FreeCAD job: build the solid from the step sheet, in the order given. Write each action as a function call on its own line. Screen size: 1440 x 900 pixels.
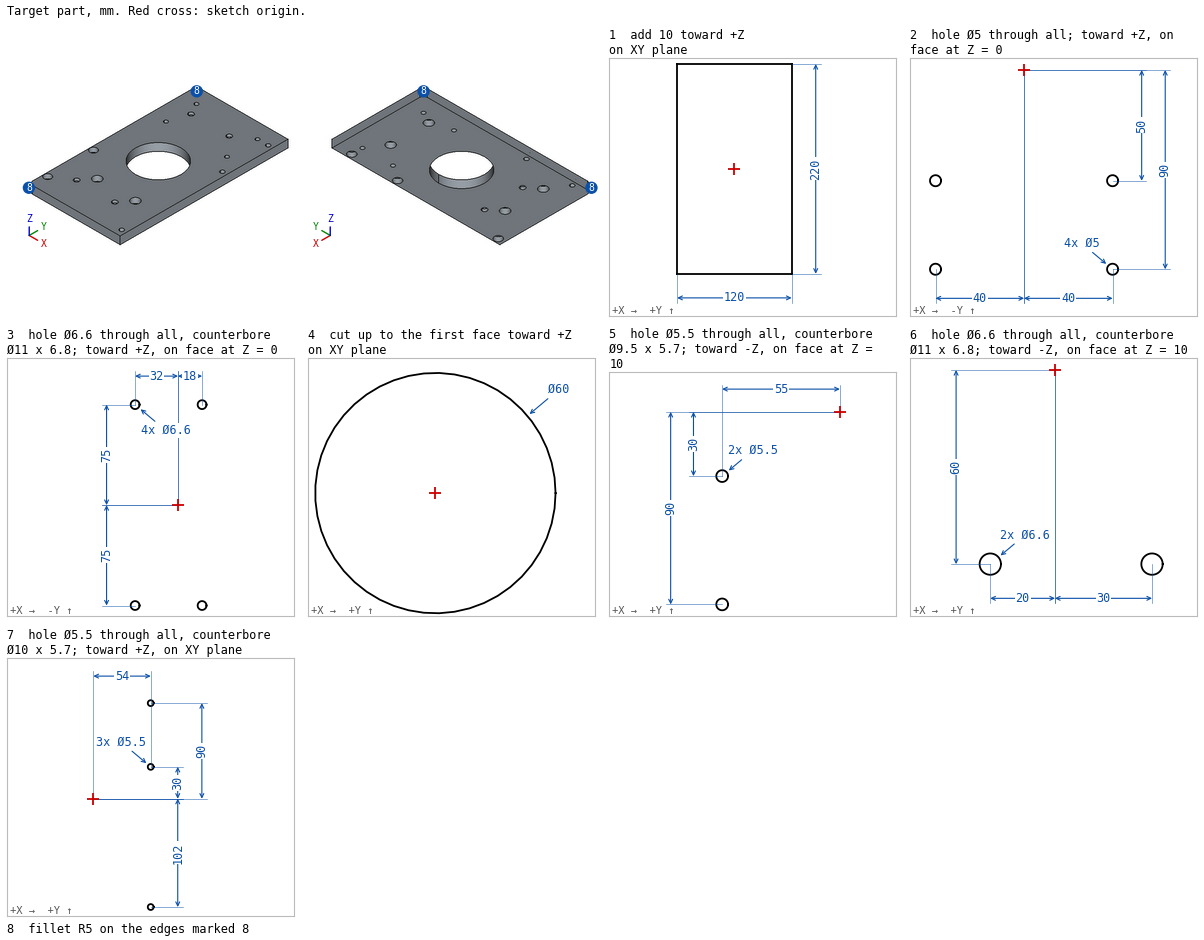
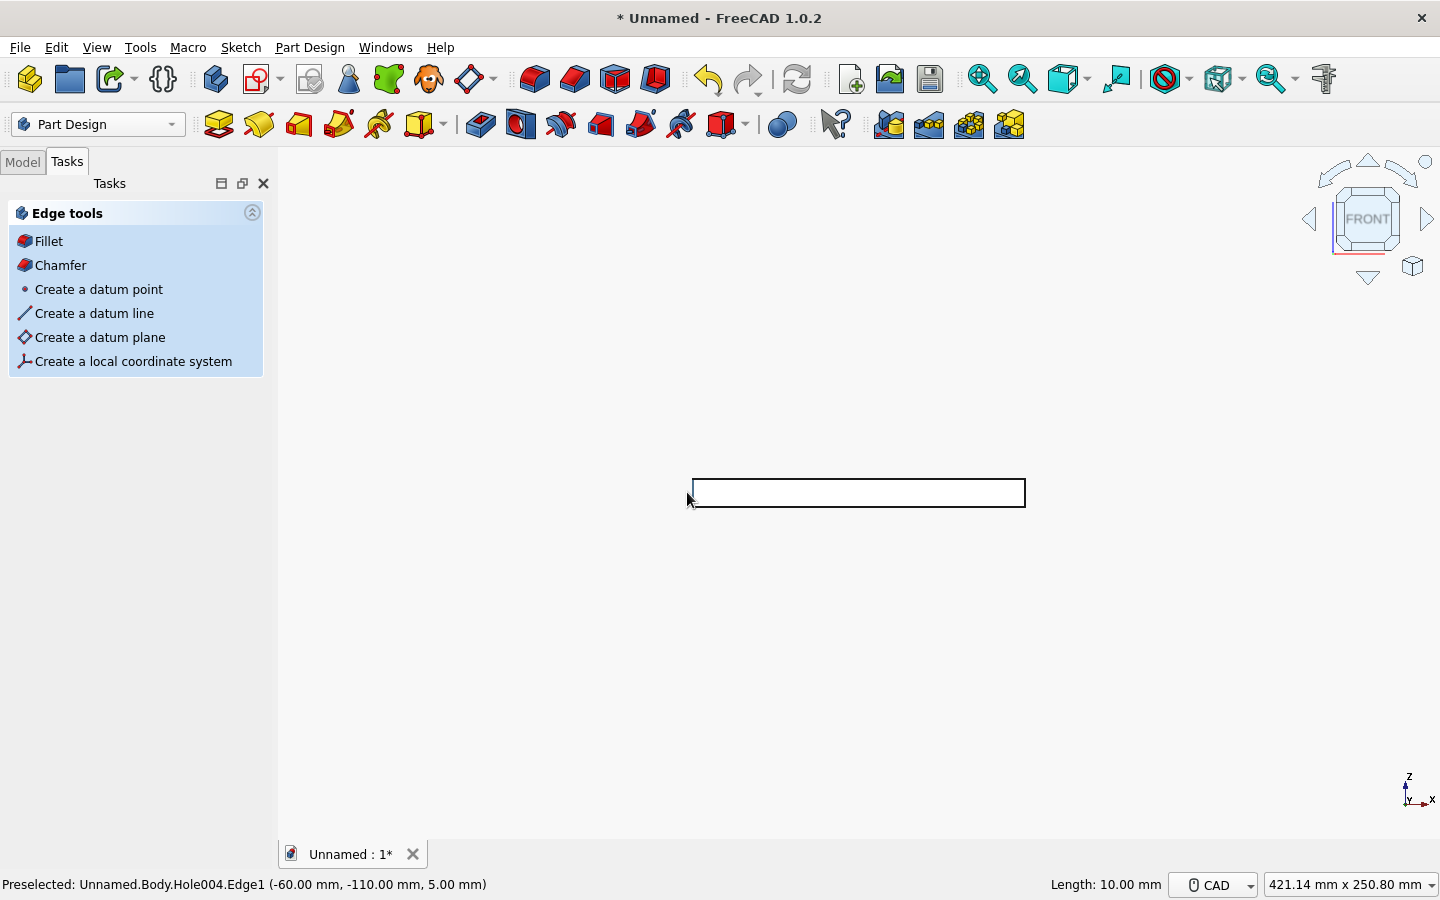
key(3)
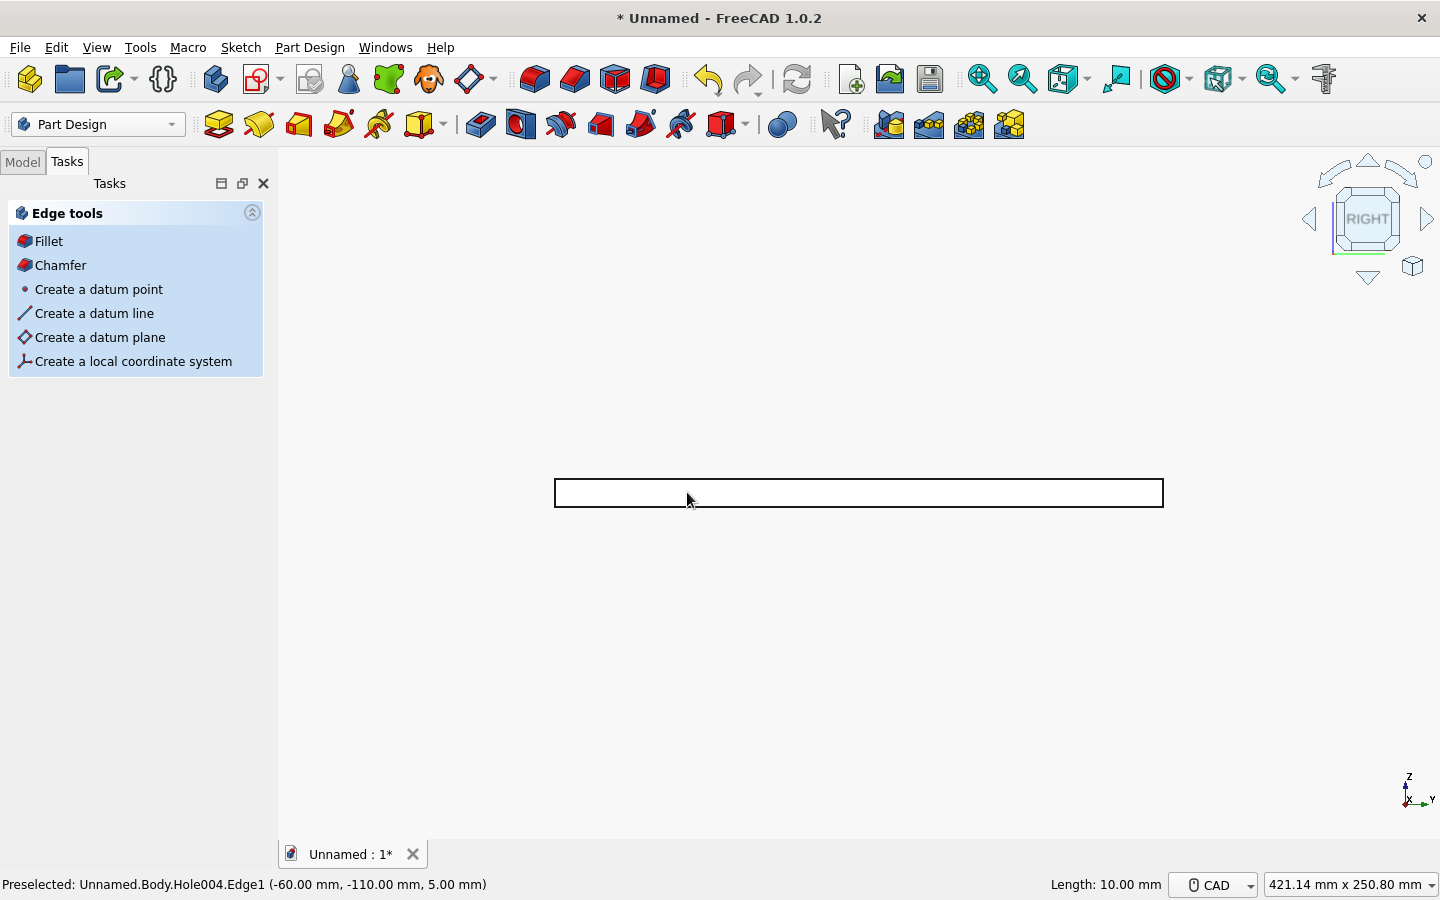
key(5)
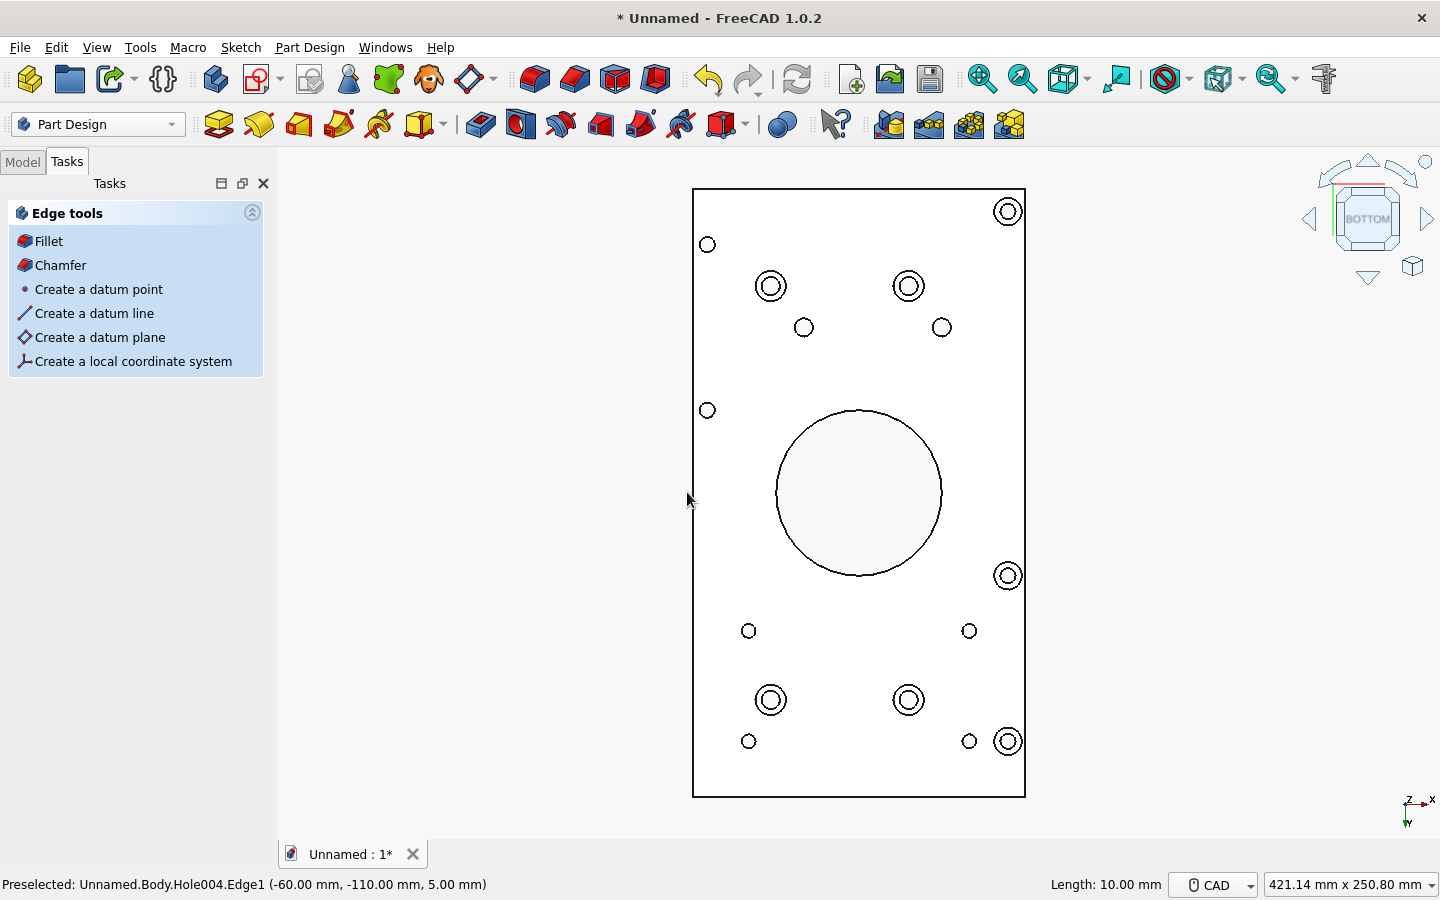
key(4)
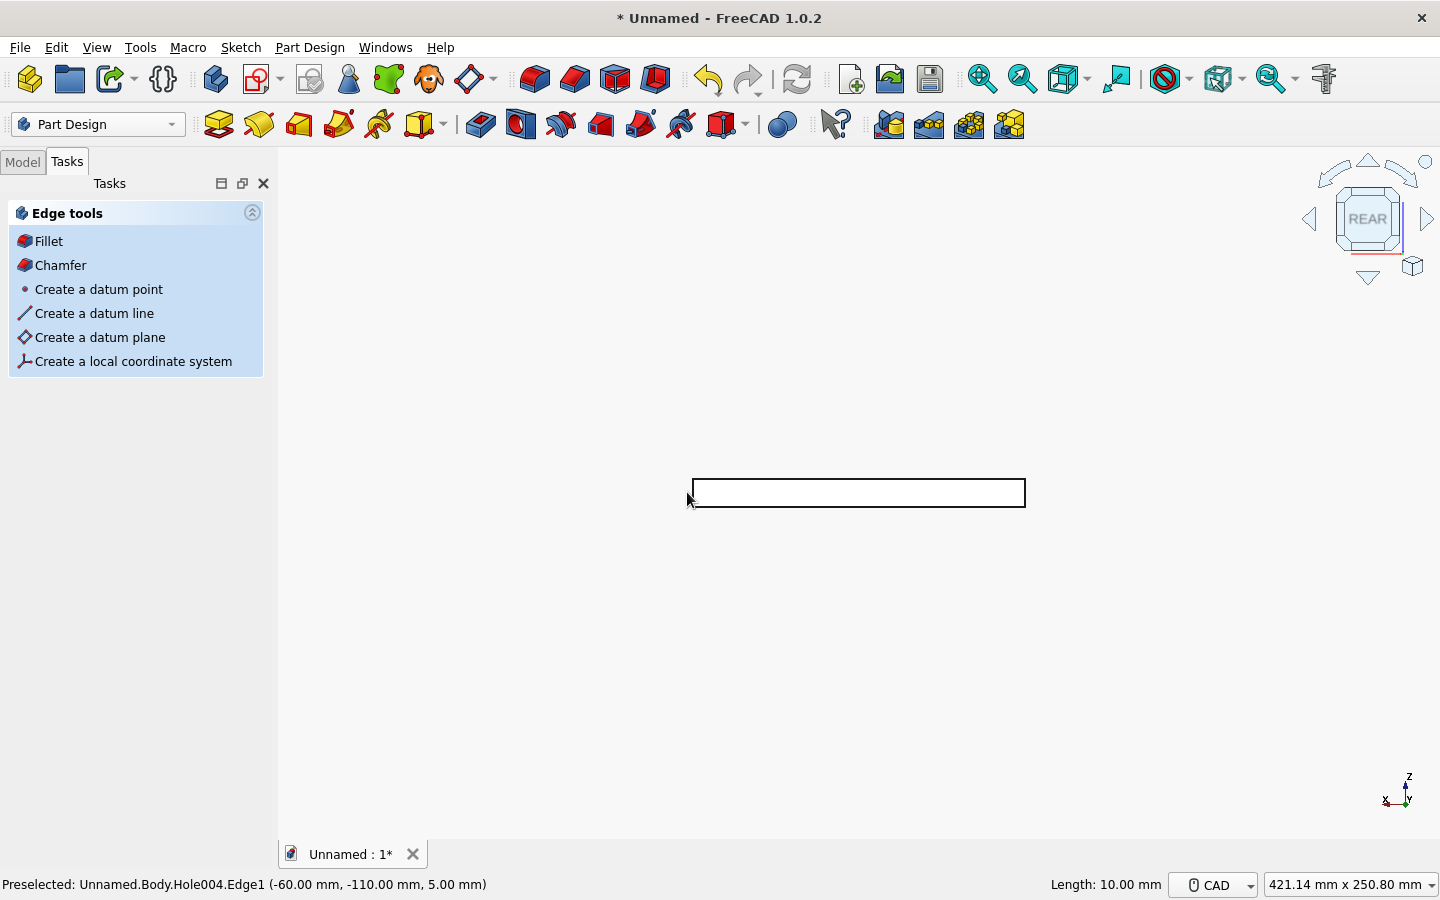
key(v)
key(f)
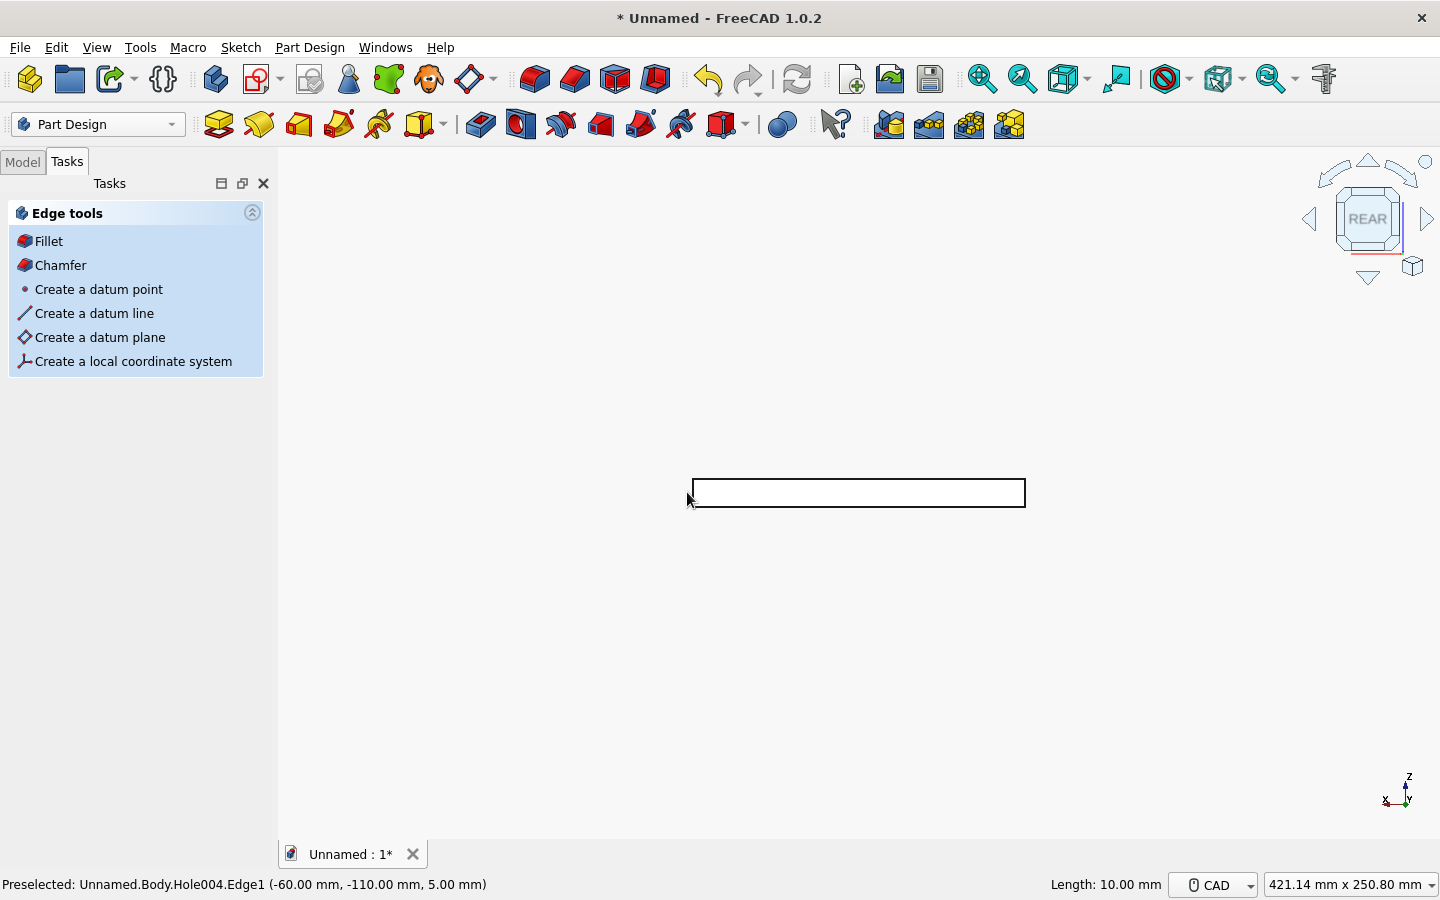
click(1025, 492, ctrl)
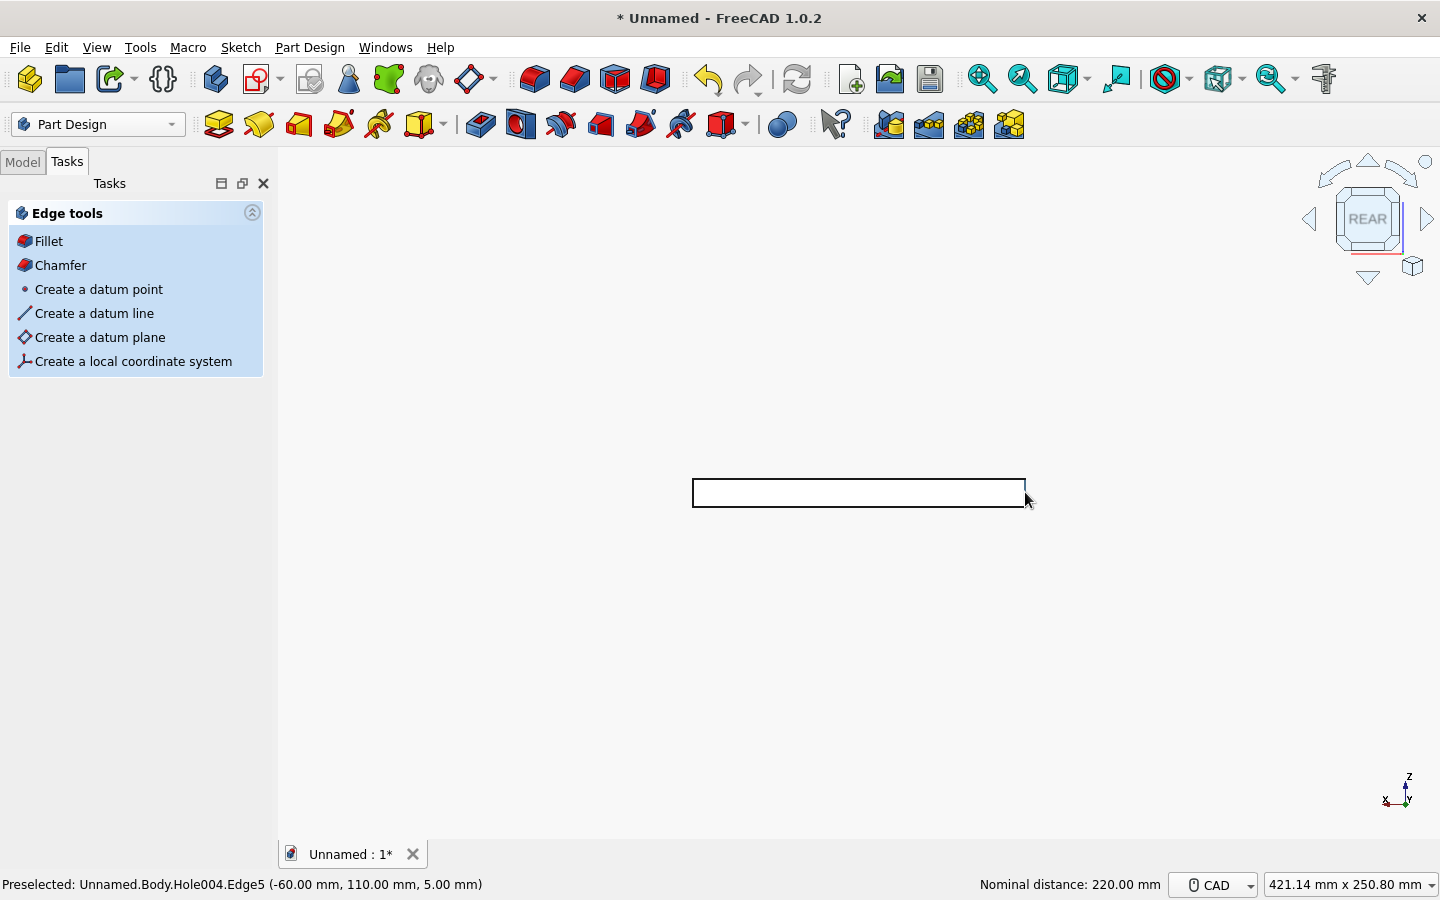
click(536, 80)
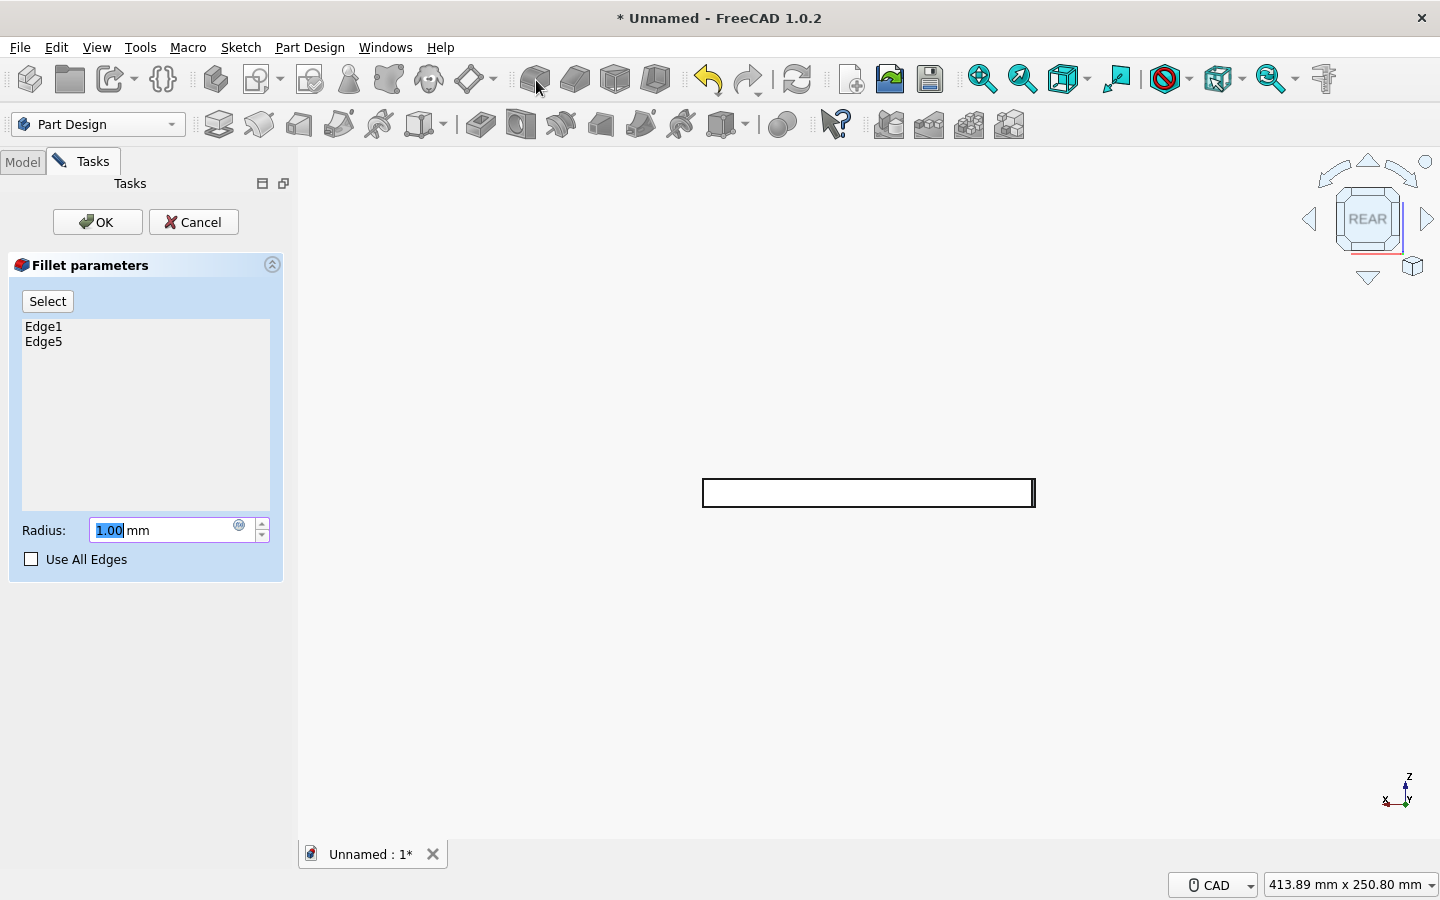
text(5)
key(Tab)